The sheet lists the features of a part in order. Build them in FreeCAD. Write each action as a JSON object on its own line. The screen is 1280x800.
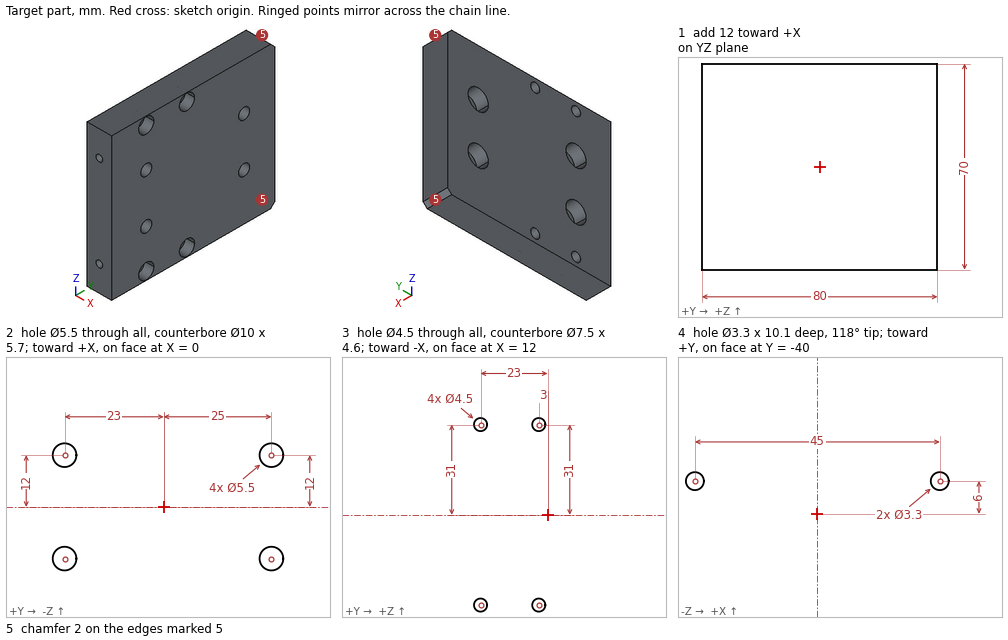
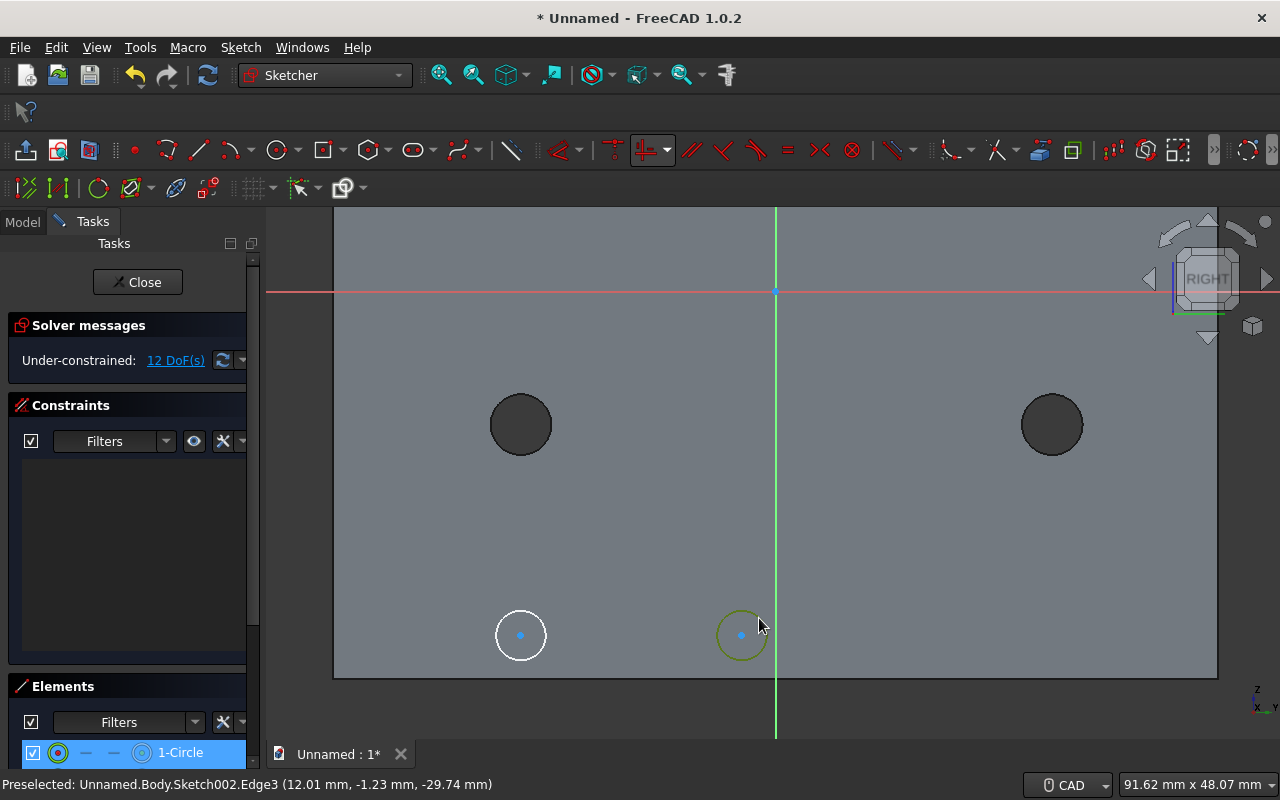
{"action": "left_click", "coordinate": [538, 618]}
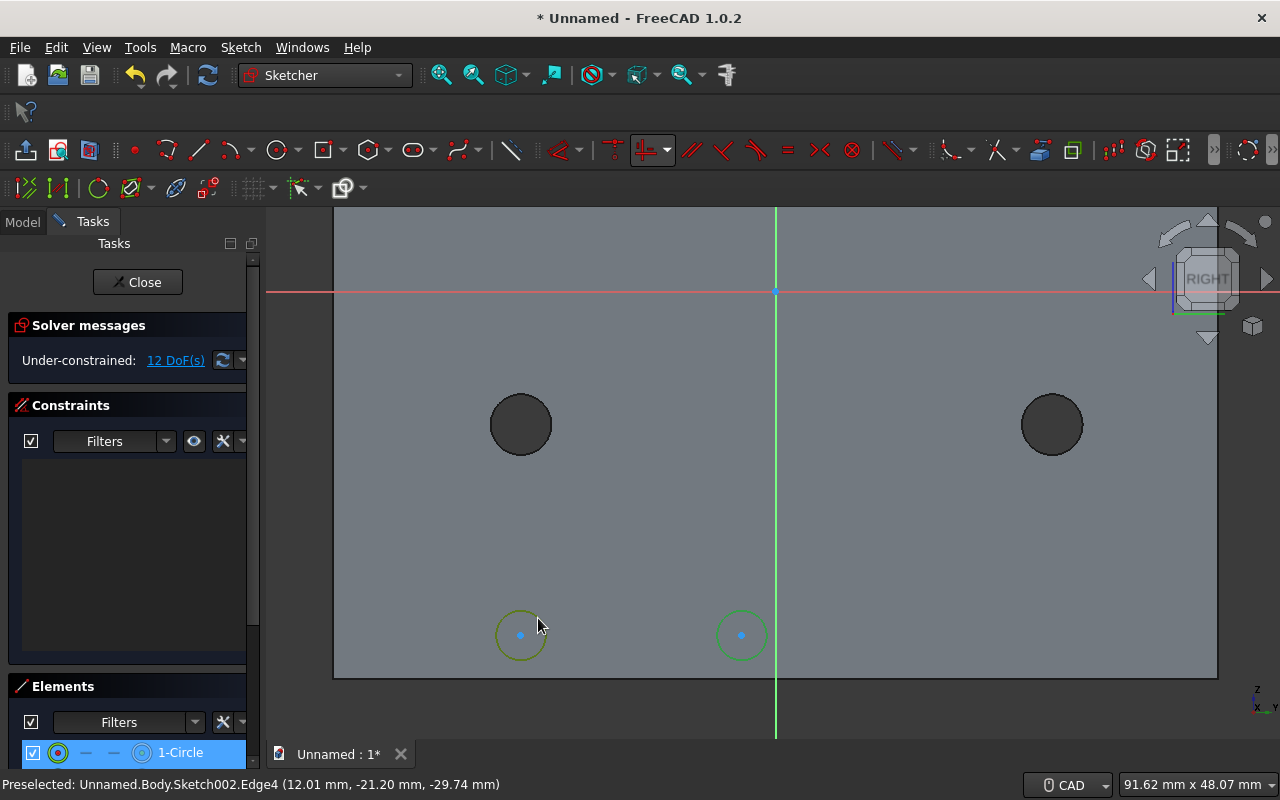
{"action": "left_click", "coordinate": [788, 150]}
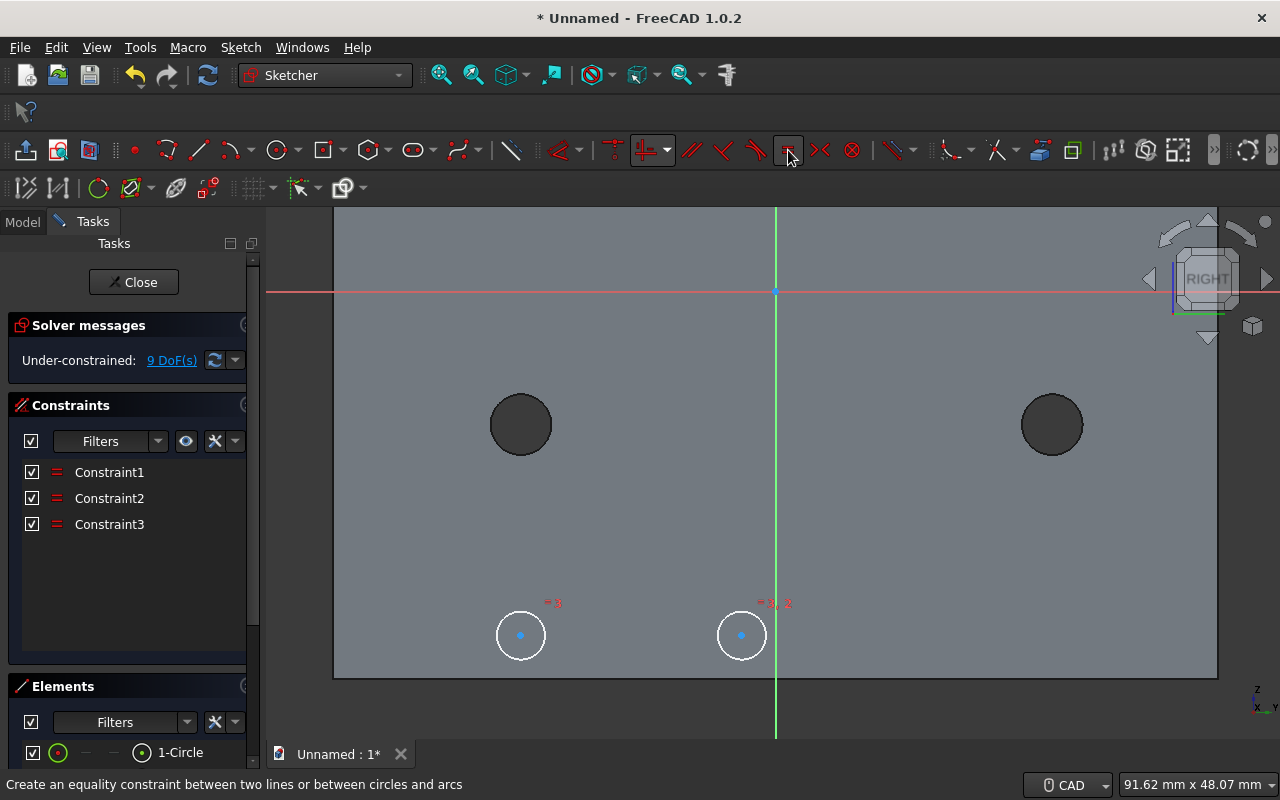
{"action": "scroll", "coordinate": [761, 621], "scroll_direction": "down", "scroll_amount": 4}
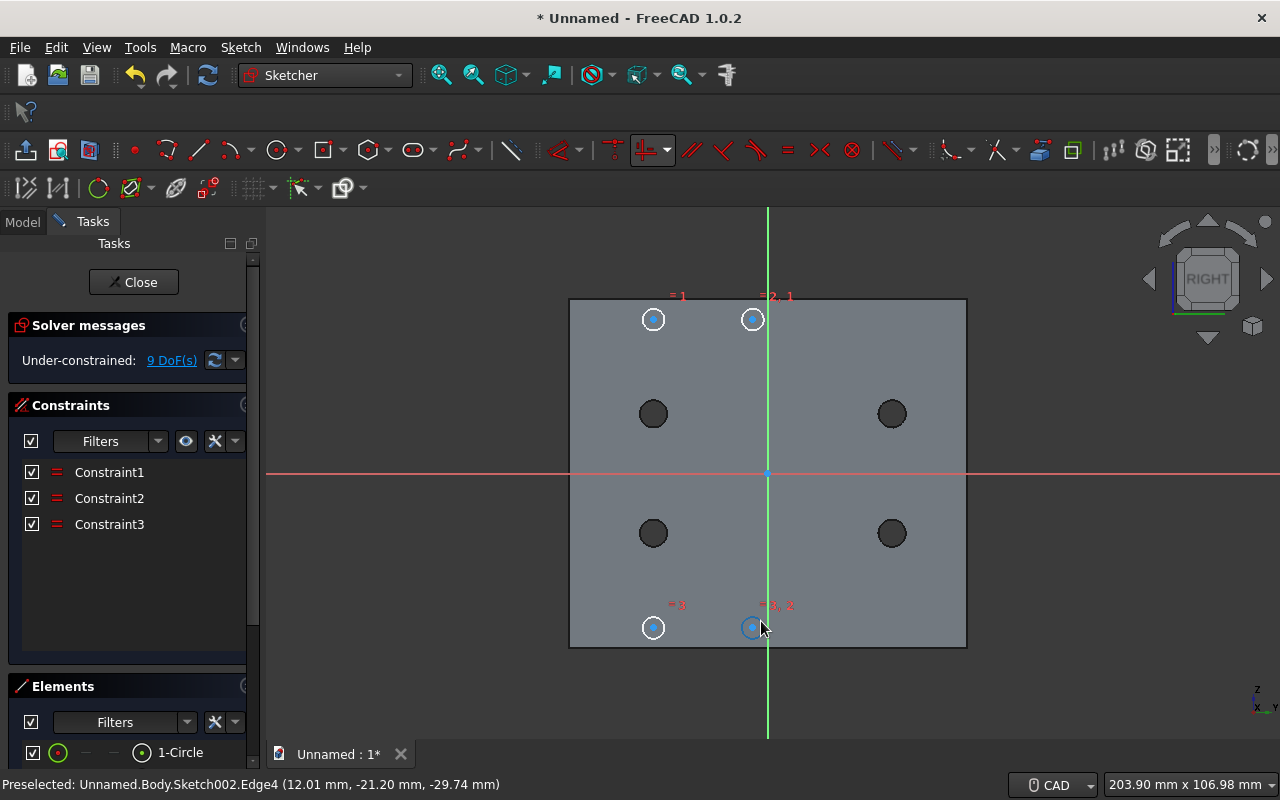
{"action": "left_click", "coordinate": [753, 320]}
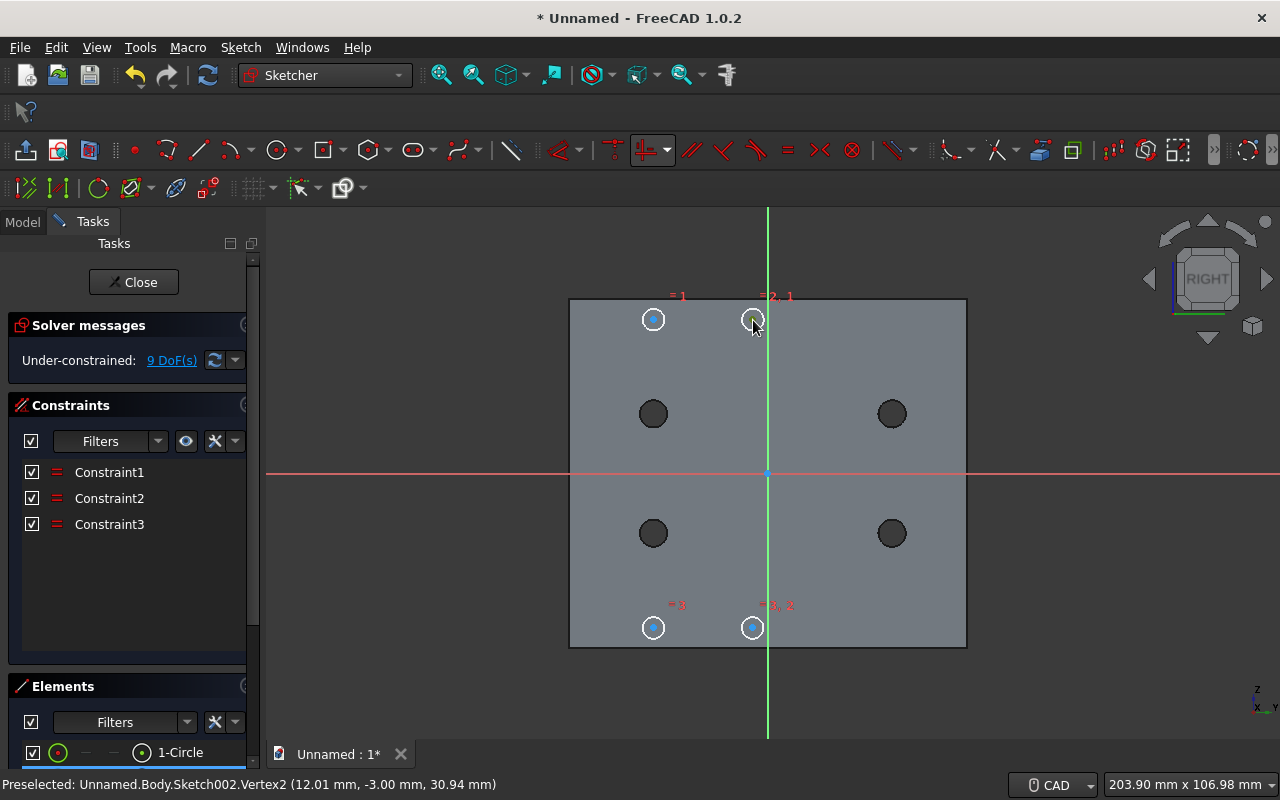
{"action": "left_click", "coordinate": [753, 628]}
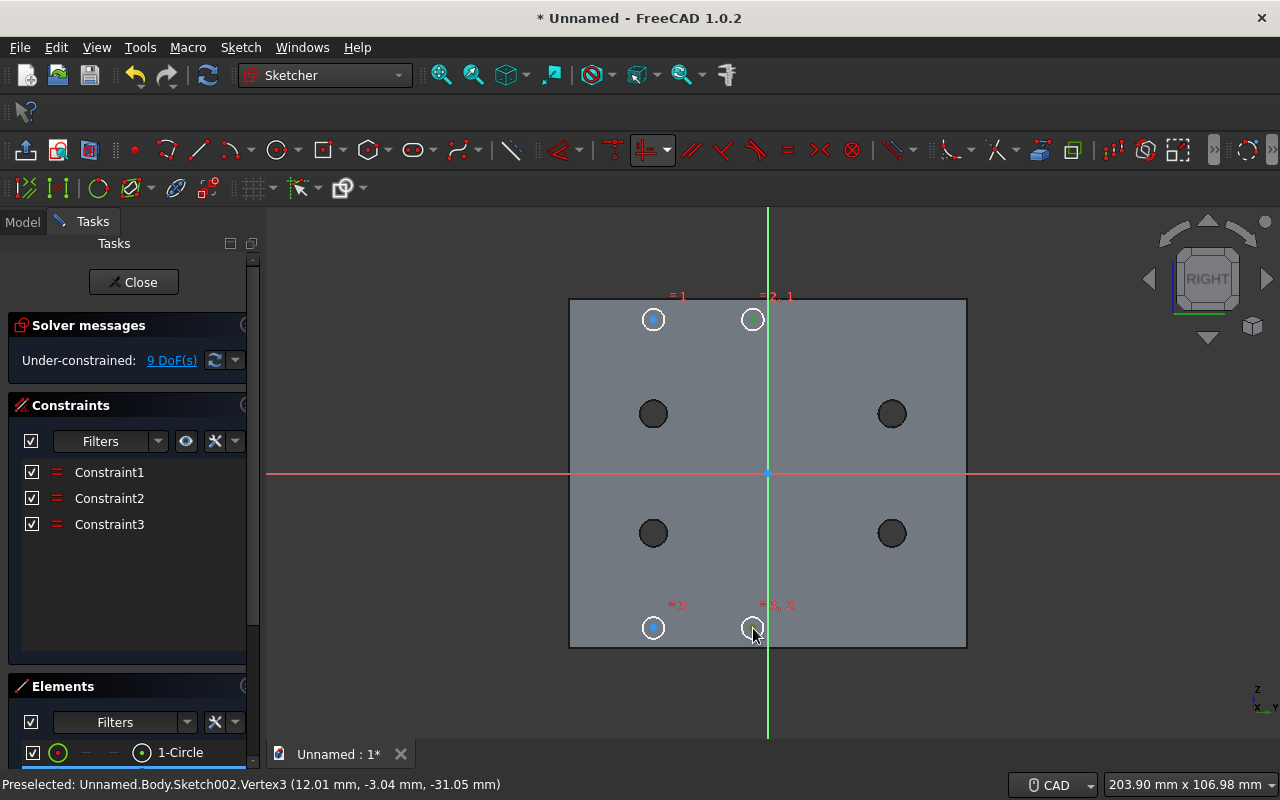
{"action": "left_click", "coordinate": [353, 474]}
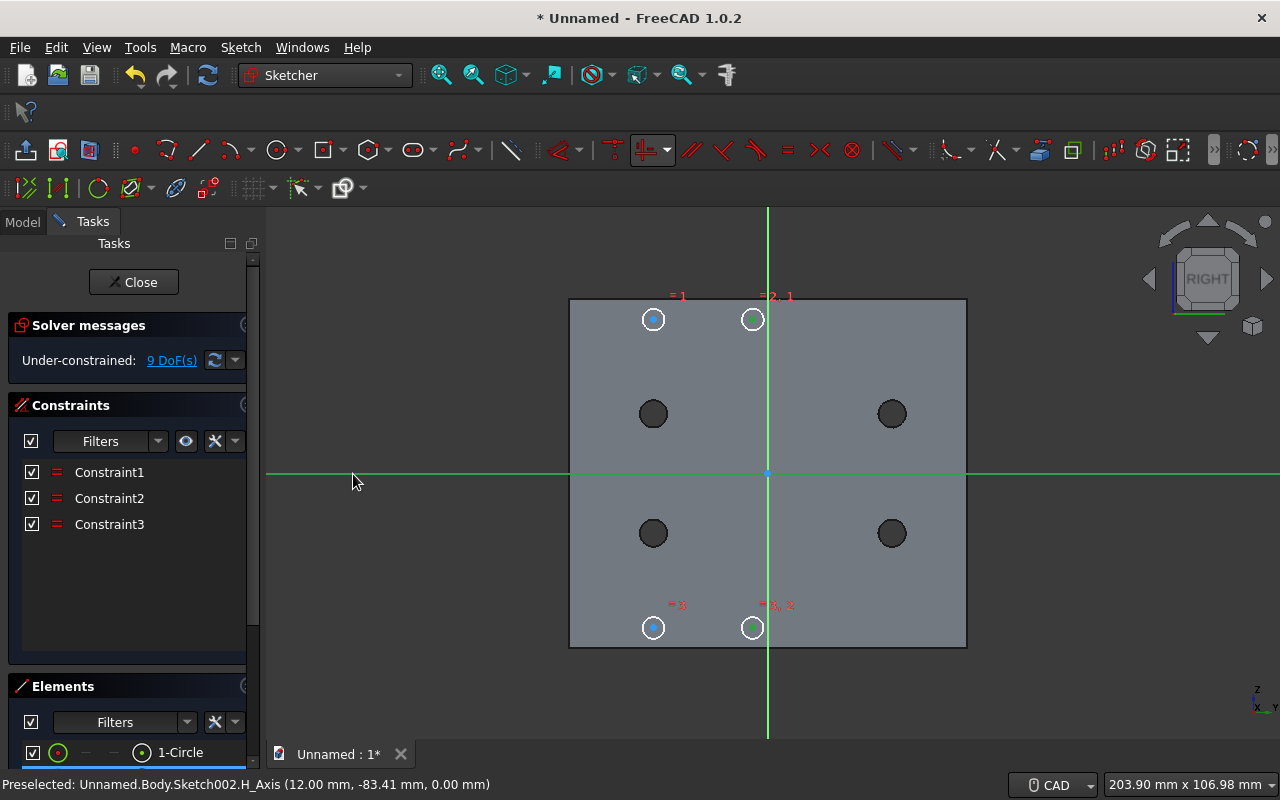
{"action": "left_click", "coordinate": [820, 150]}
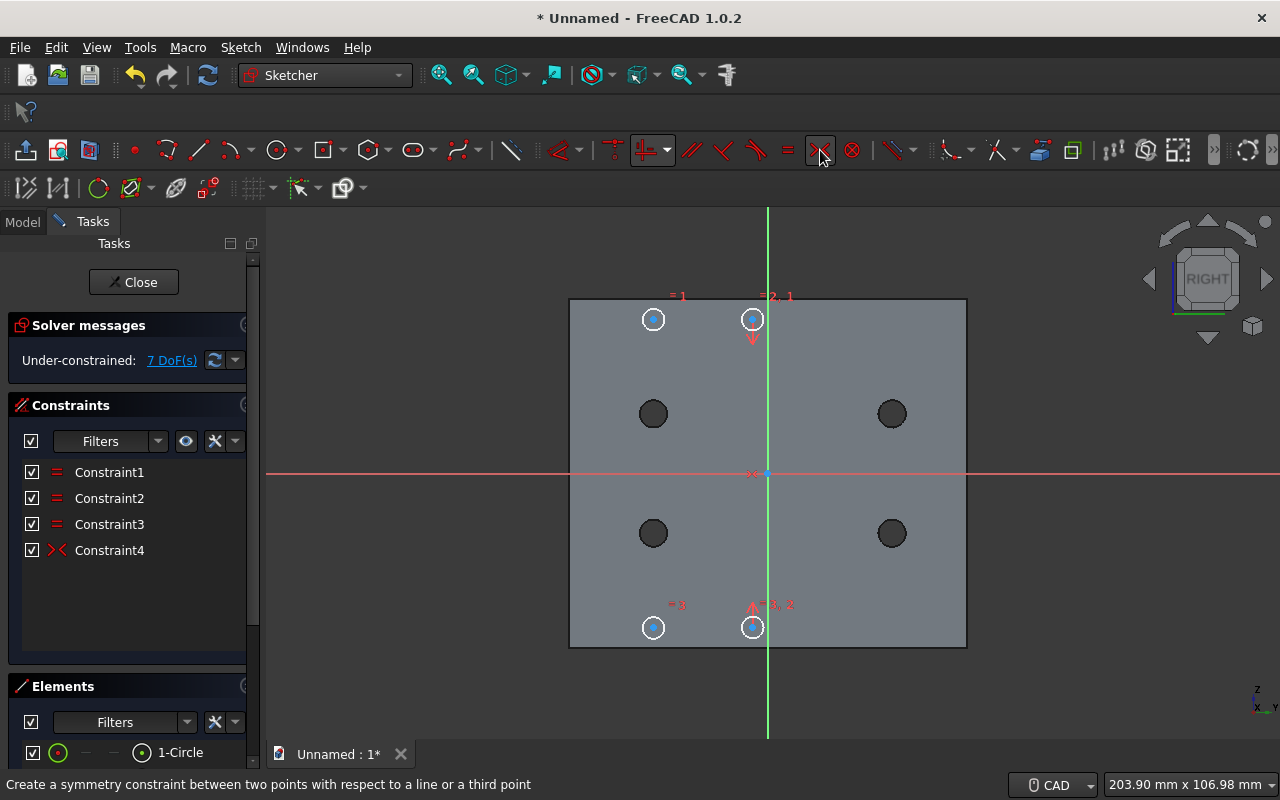
{"action": "left_click", "coordinate": [654, 320]}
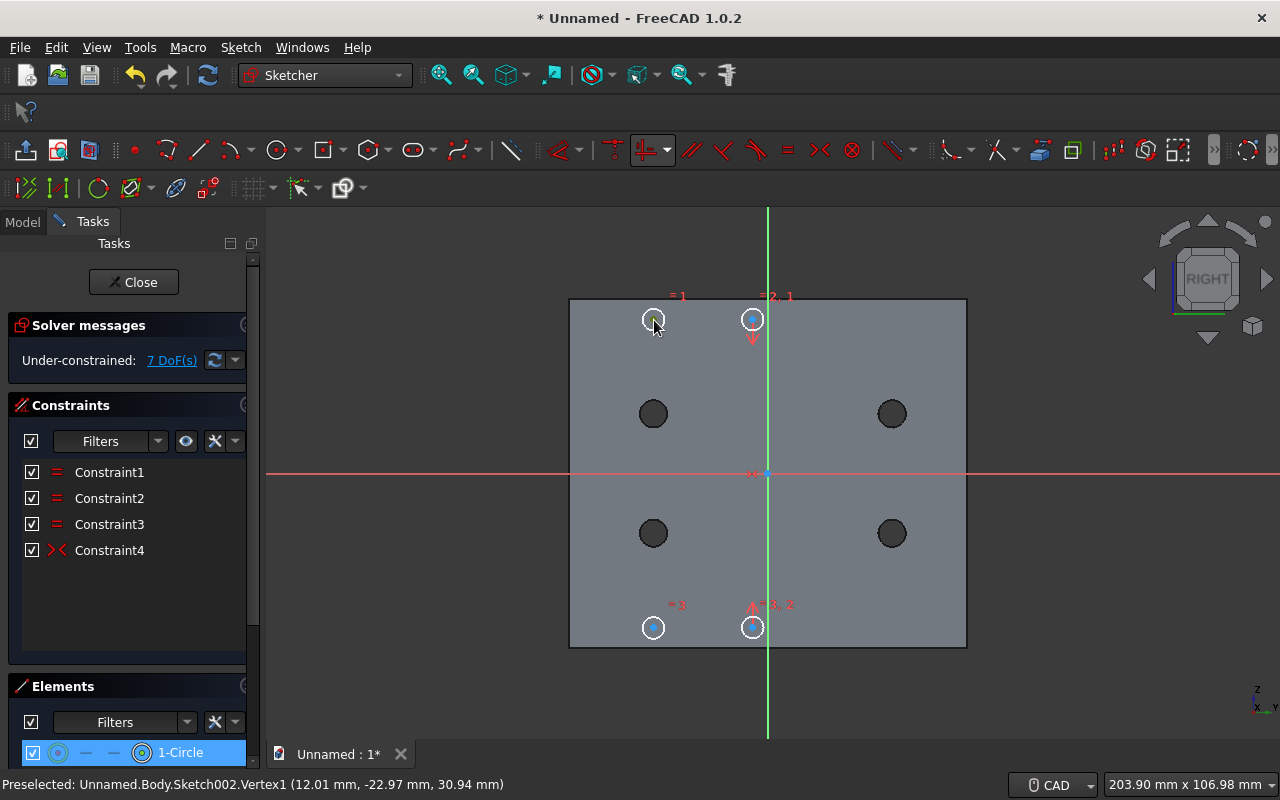
{"action": "left_click", "coordinate": [653, 628]}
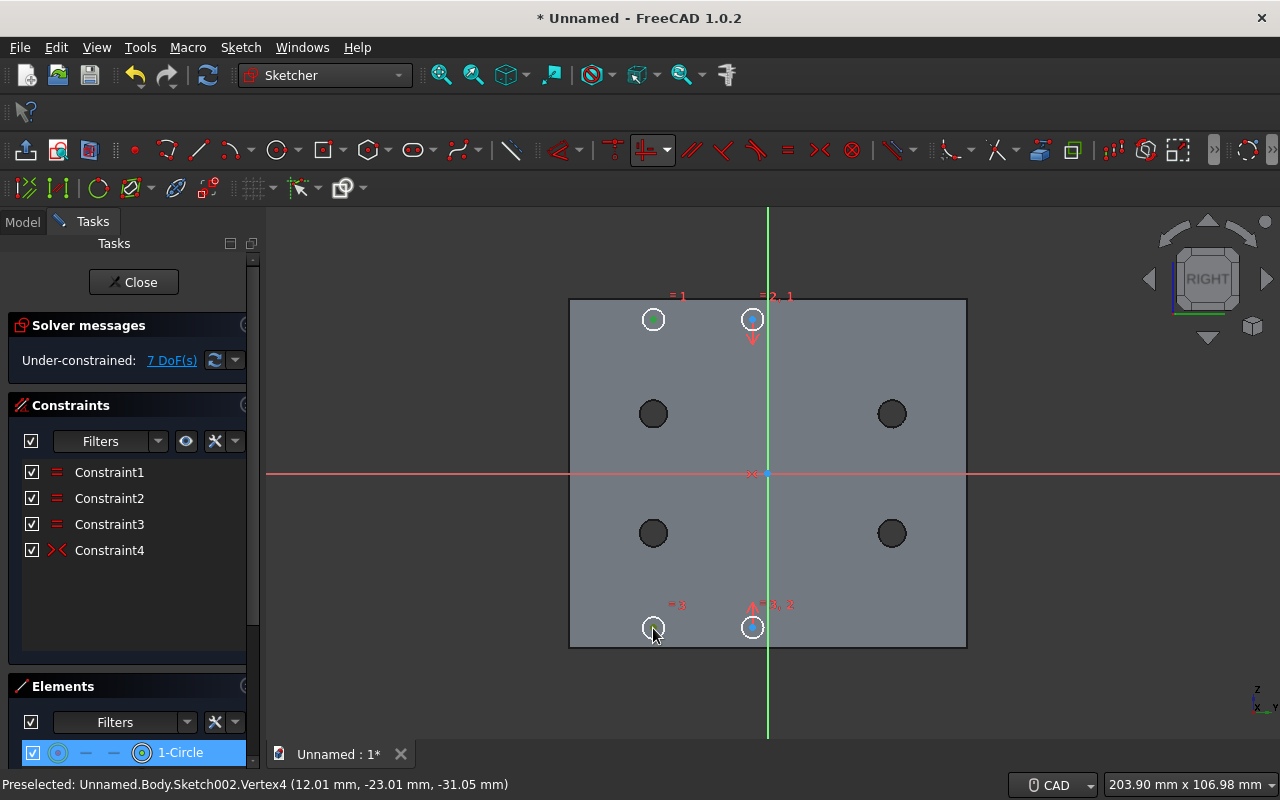
{"action": "left_click", "coordinate": [353, 474]}